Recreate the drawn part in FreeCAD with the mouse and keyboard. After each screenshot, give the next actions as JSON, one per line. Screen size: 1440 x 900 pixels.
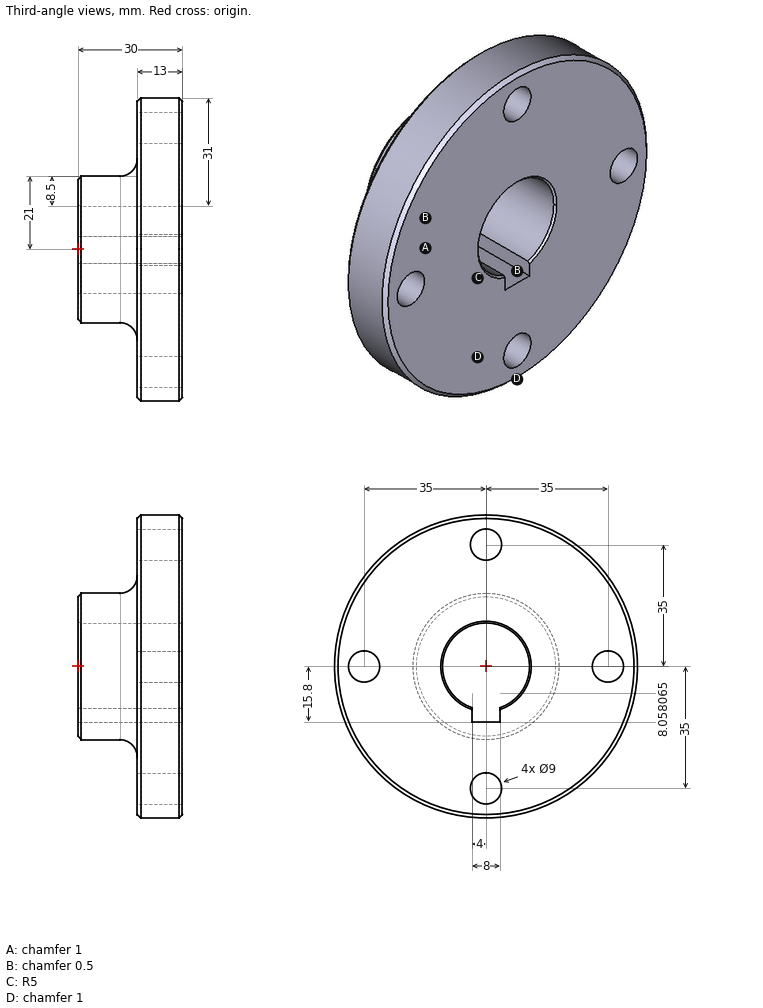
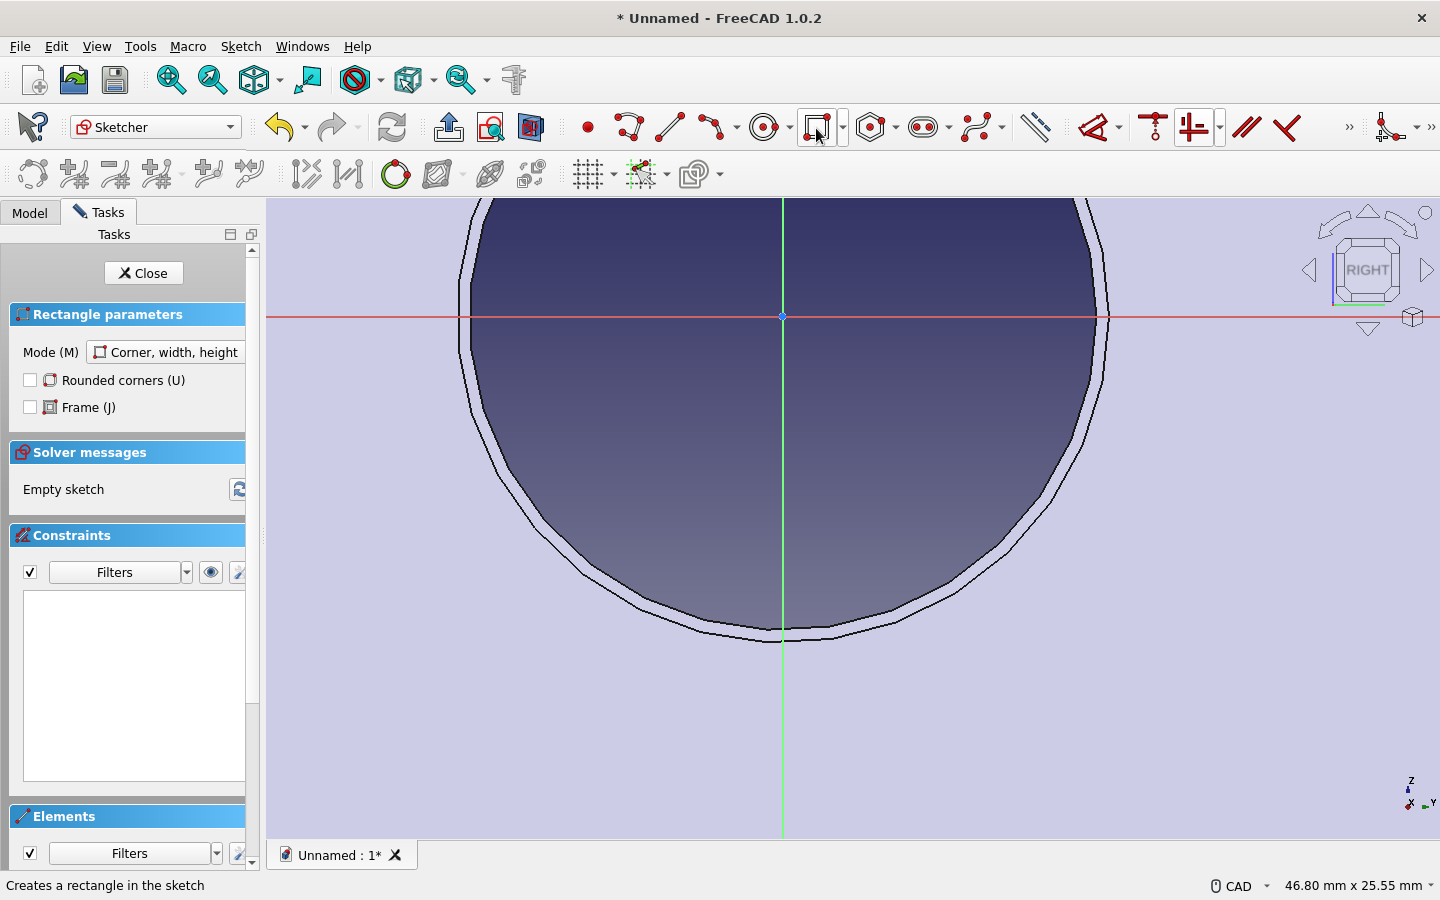
{"action": "left_click", "coordinate": [683, 511]}
{"action": "mouse_move", "coordinate": [883, 713]}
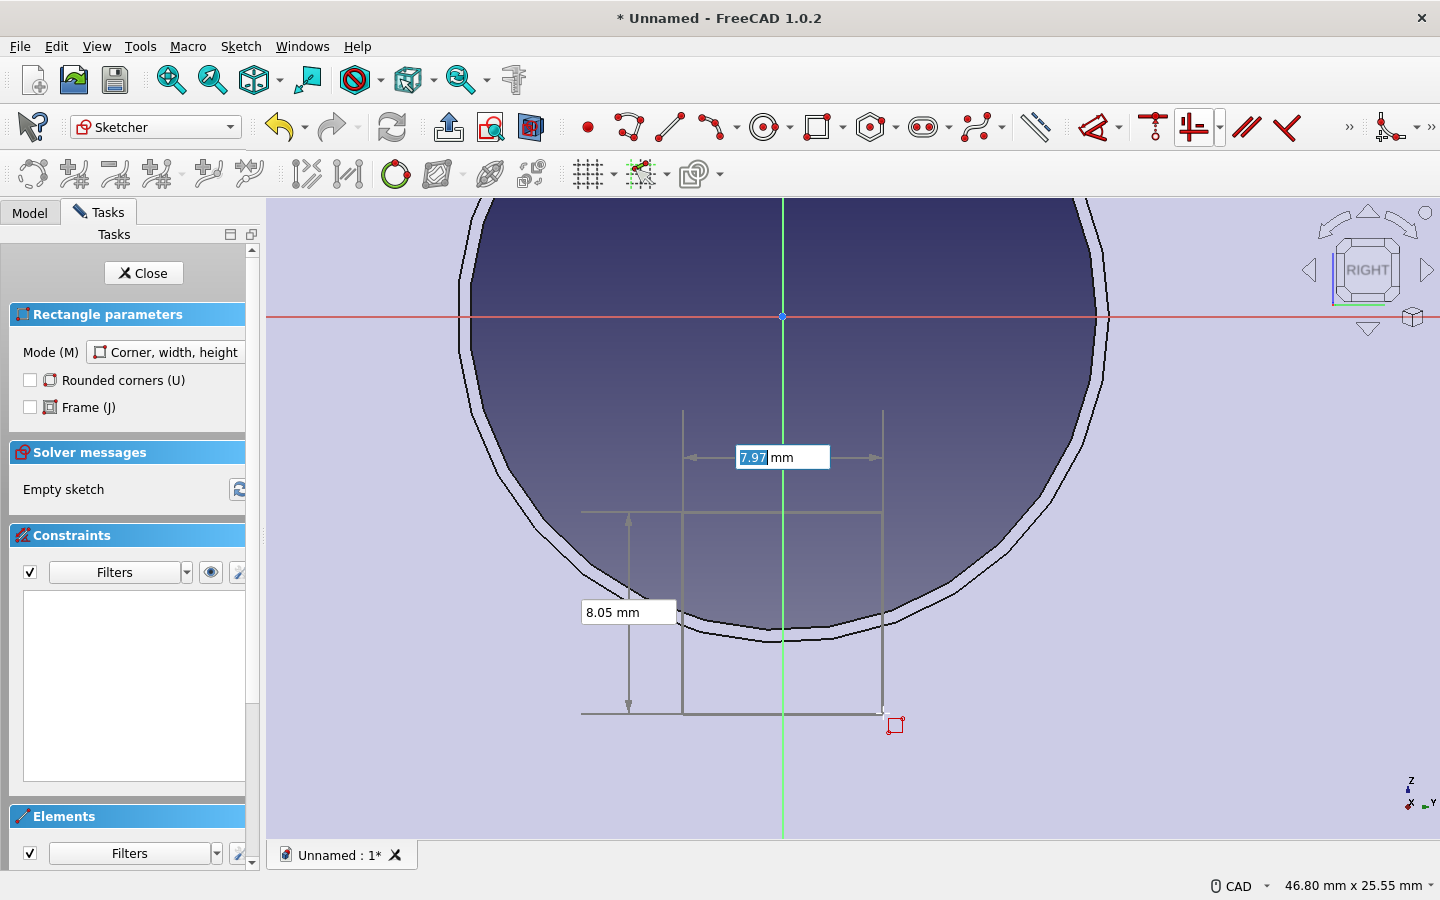
{"action": "type", "text": "8"}
{"action": "key", "text": "Tab"}
{"action": "type", "text": "8.058065"}
{"action": "key", "text": "Return"}
{"action": "key", "text": "Escape"}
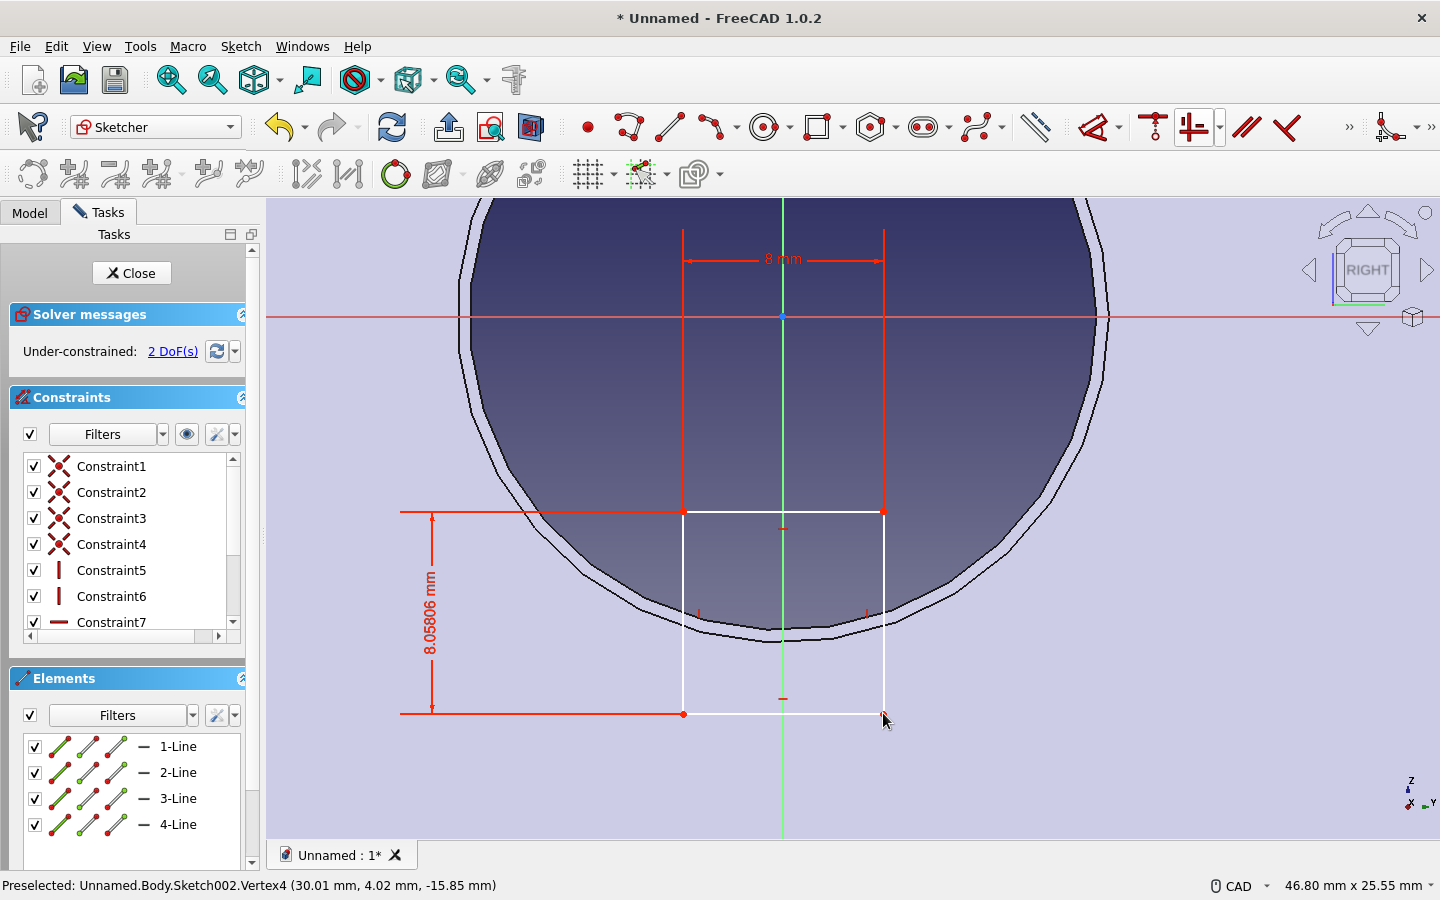
{"action": "left_click", "coordinate": [1092, 128]}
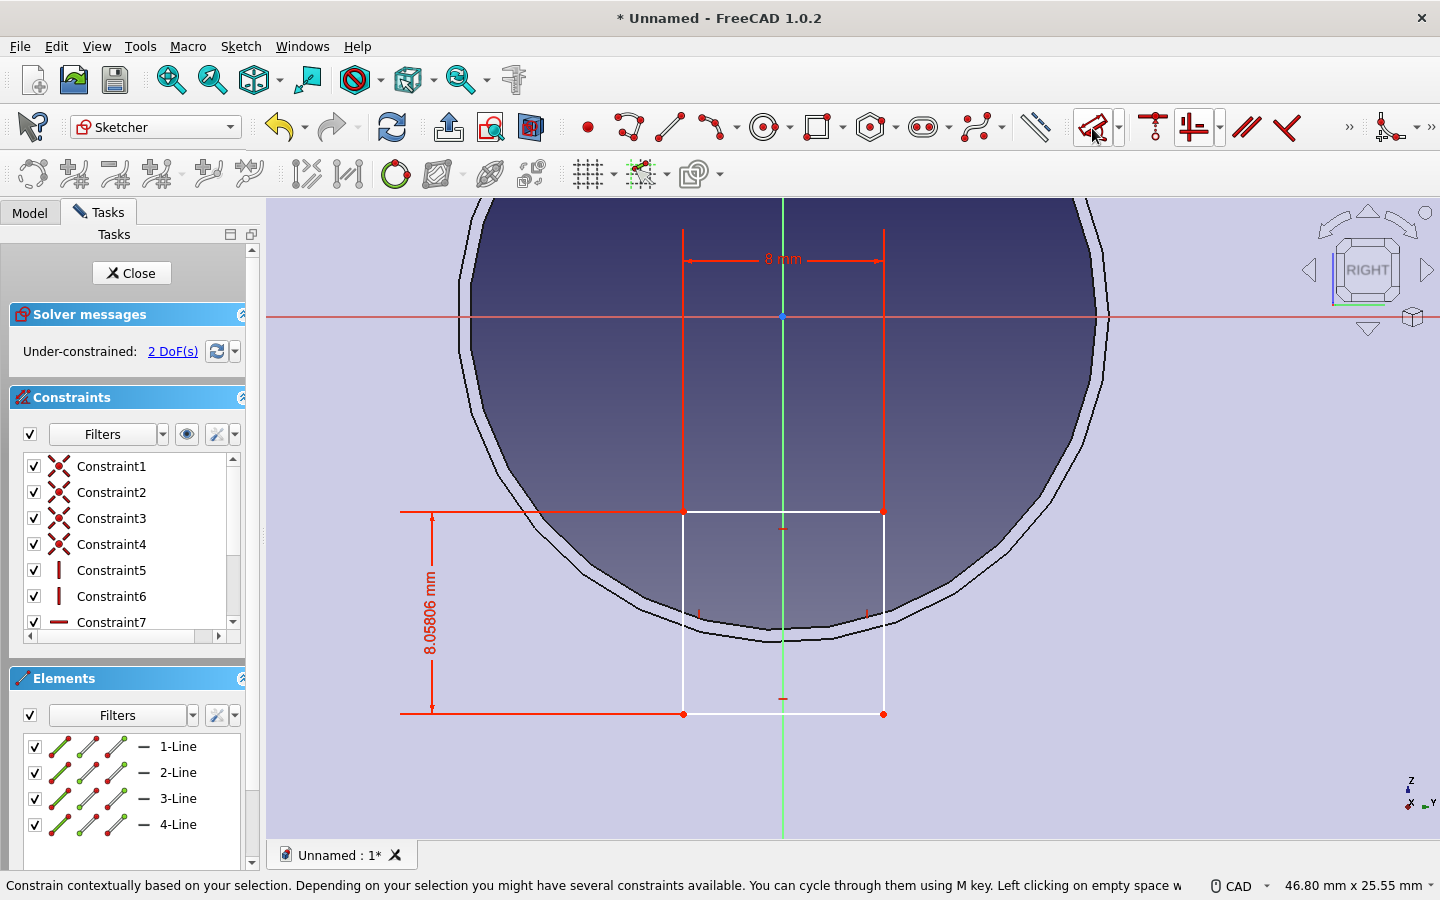
{"action": "left_click", "coordinate": [683, 512]}
{"action": "left_click", "coordinate": [733, 283]}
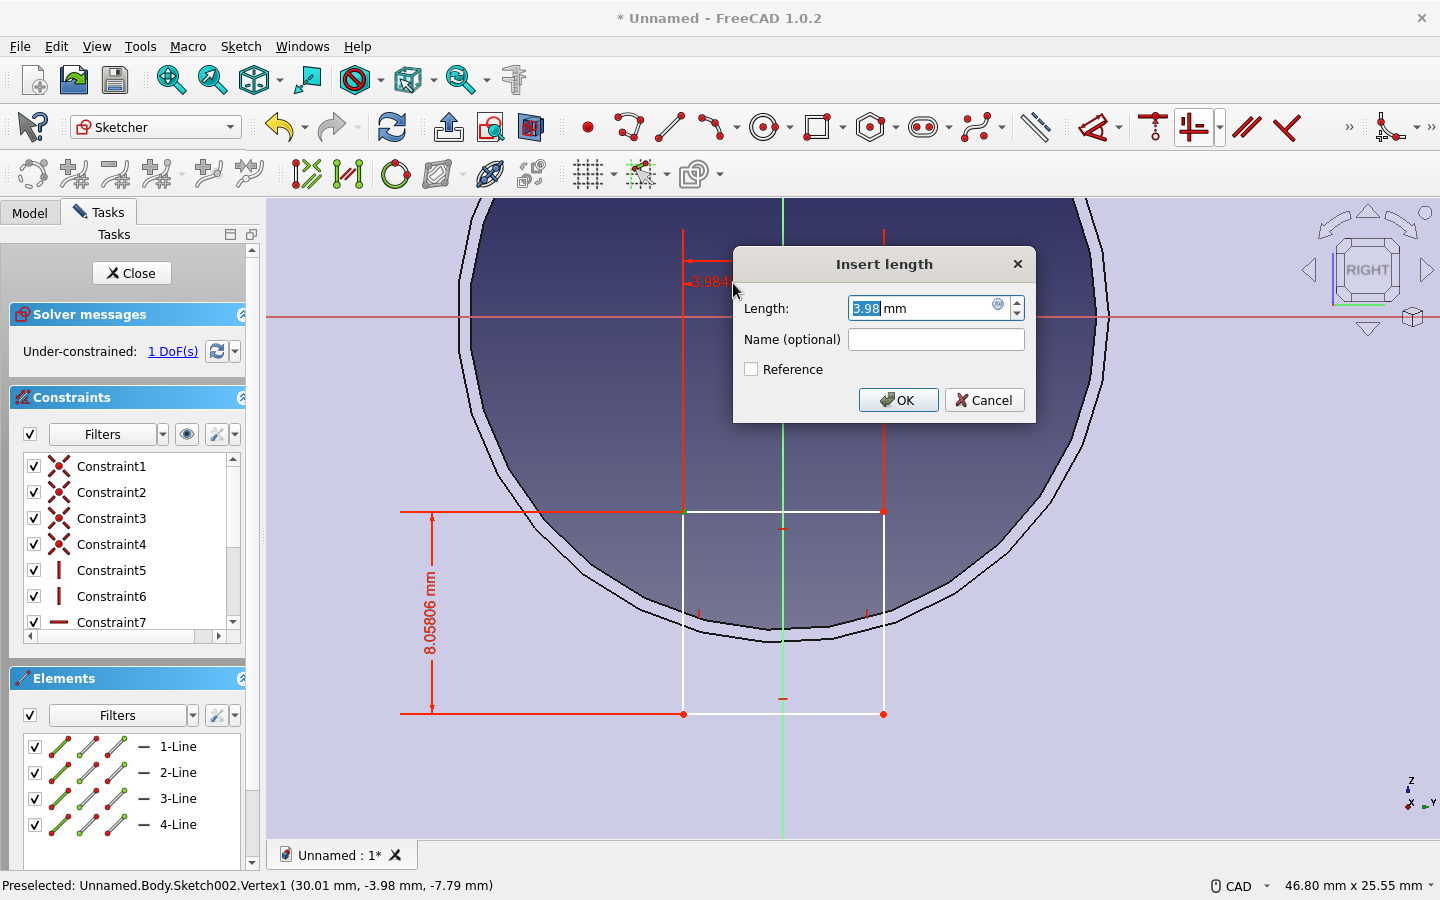
{"action": "type", "text": "4"}
{"action": "key", "text": "Return"}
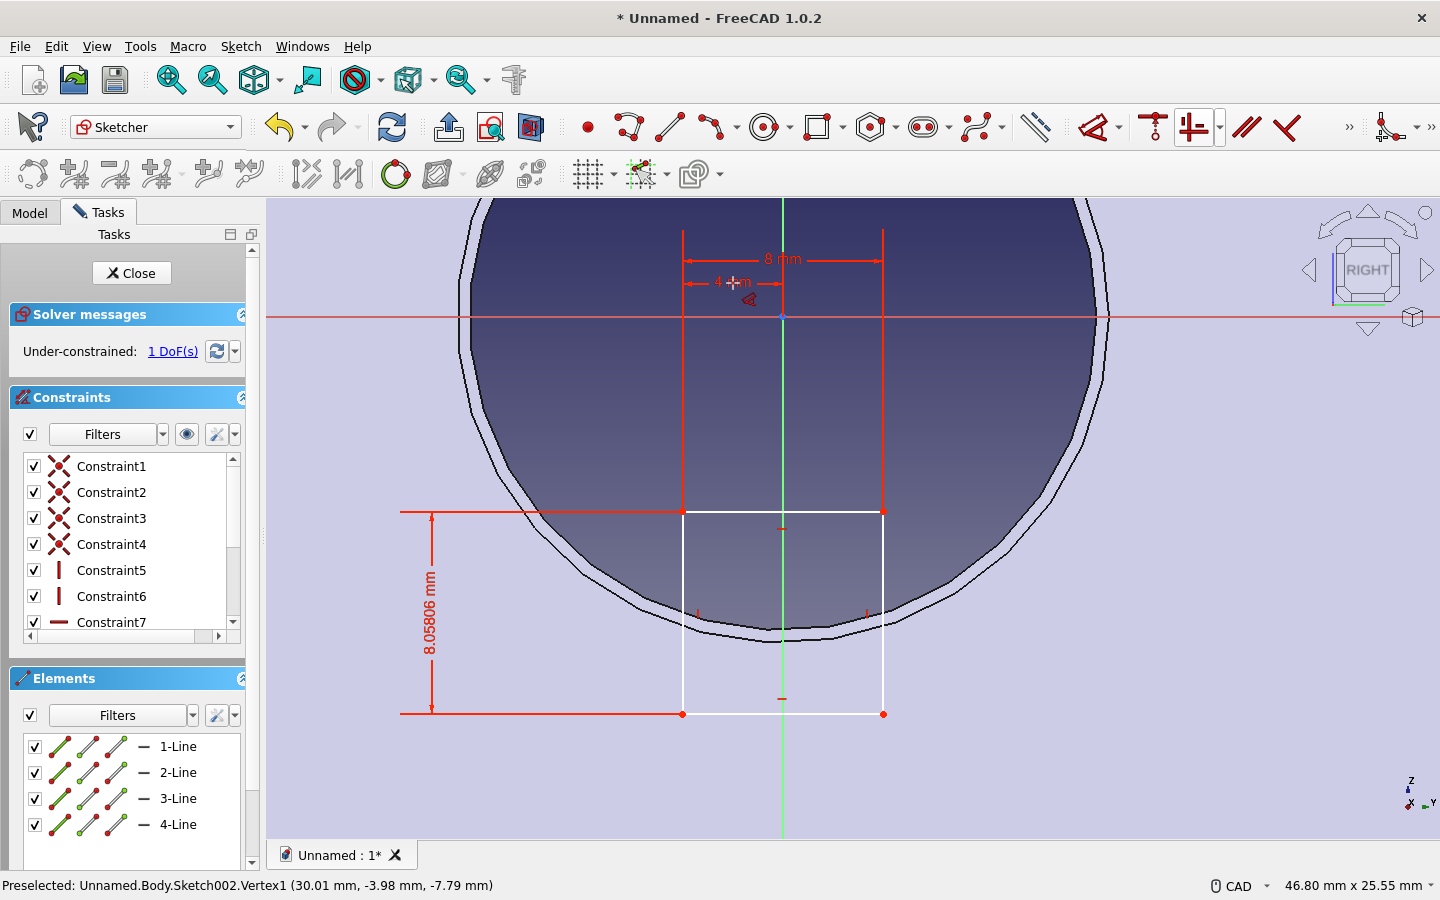
{"action": "left_click", "coordinate": [683, 714]}
{"action": "left_click", "coordinate": [649, 515]}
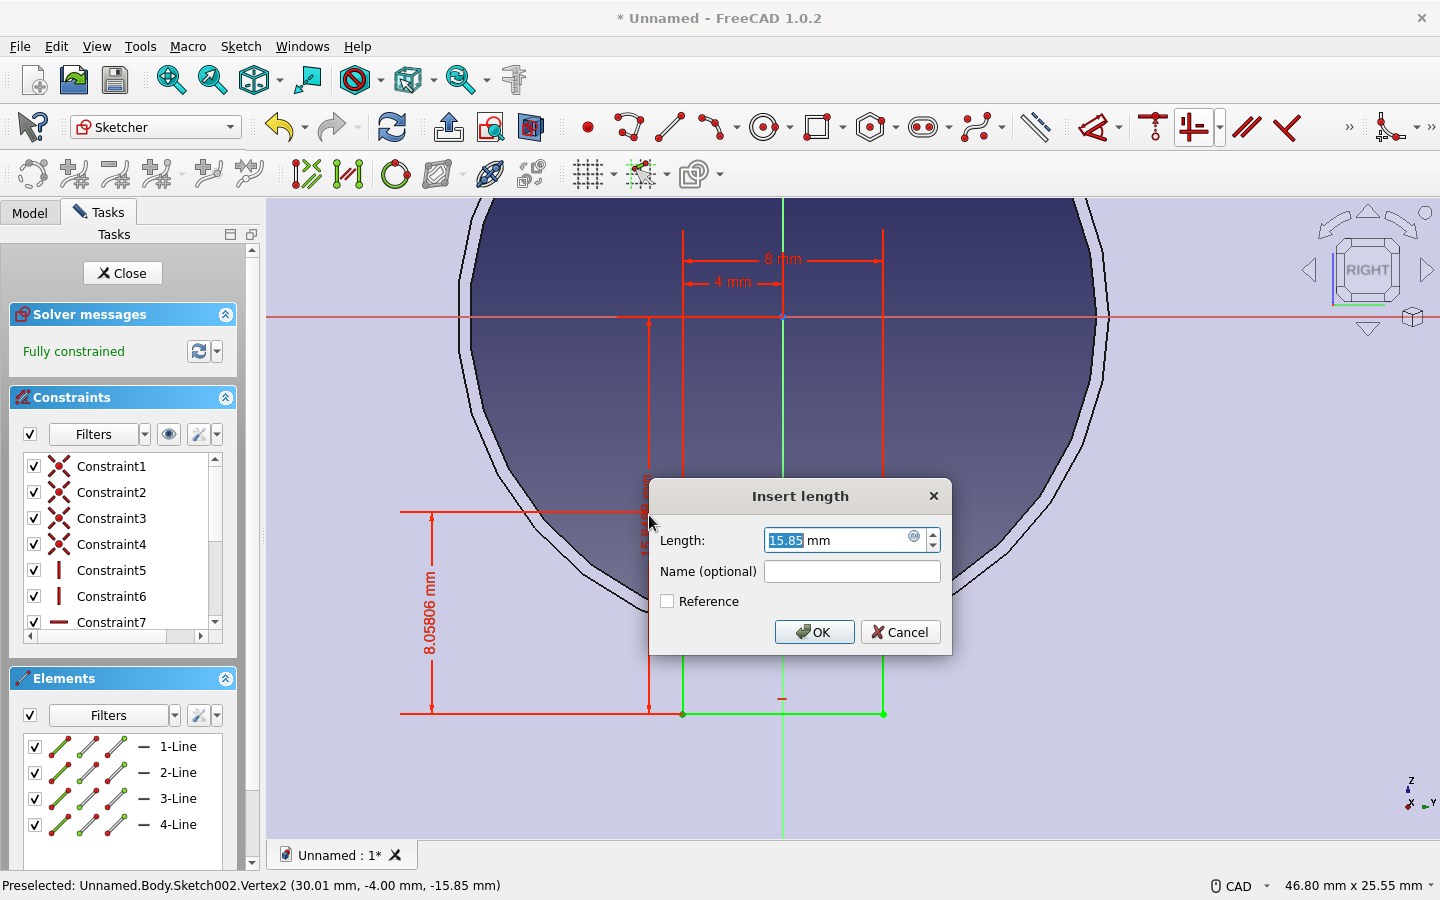
{"action": "type", "text": "15.8"}
{"action": "key", "text": "Return"}
{"action": "key", "text": "Escape"}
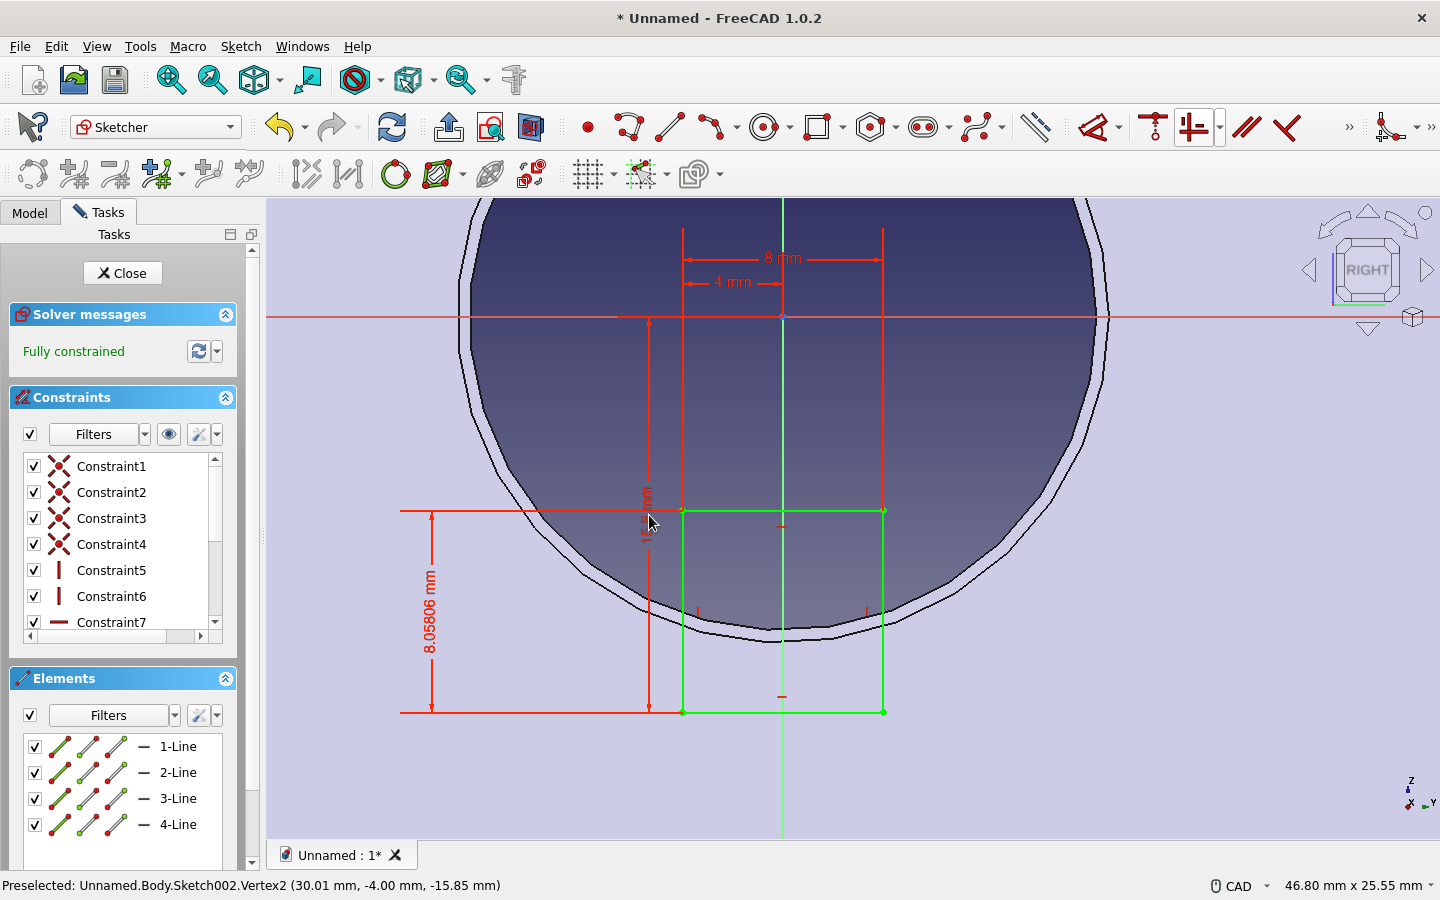
{"action": "left_click", "coordinate": [123, 273]}